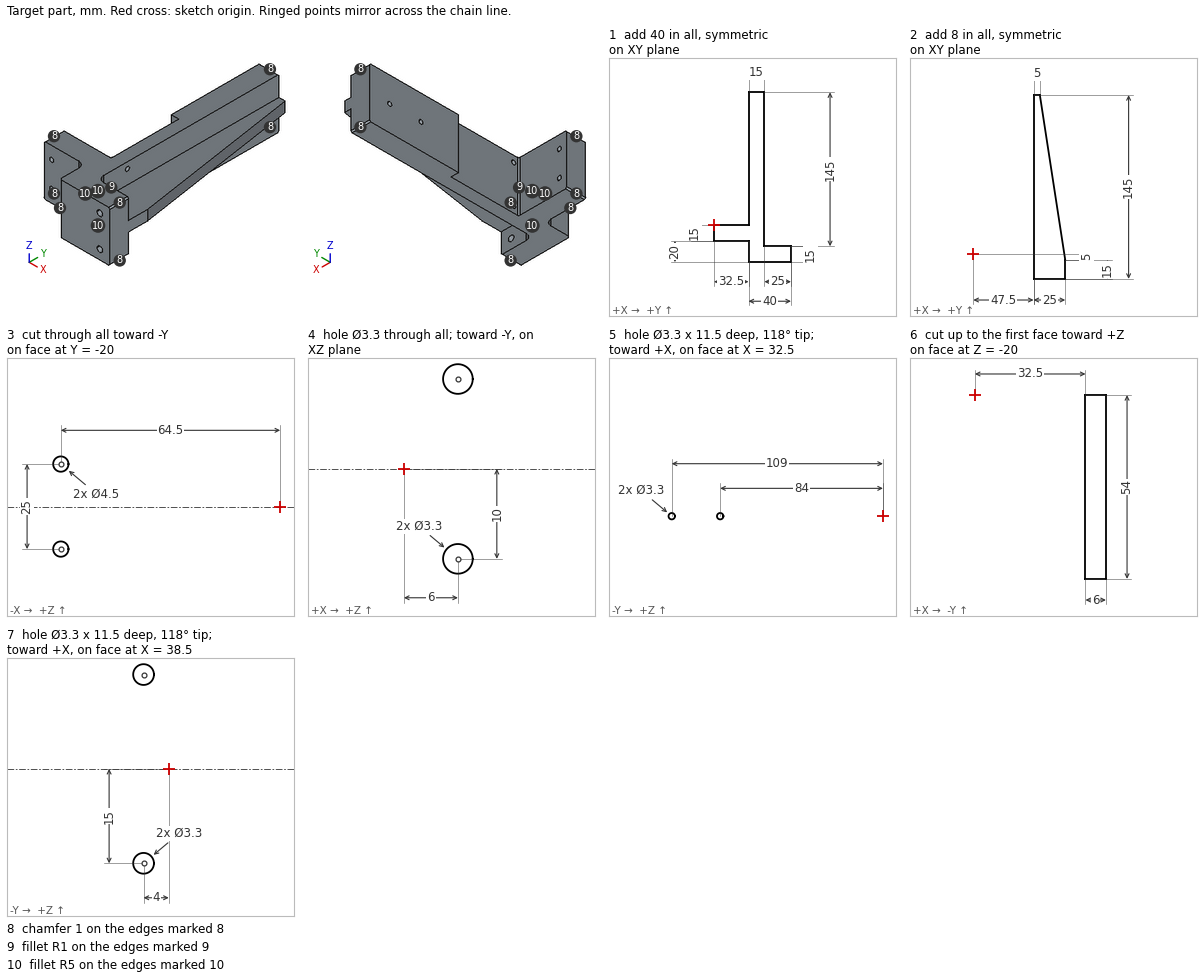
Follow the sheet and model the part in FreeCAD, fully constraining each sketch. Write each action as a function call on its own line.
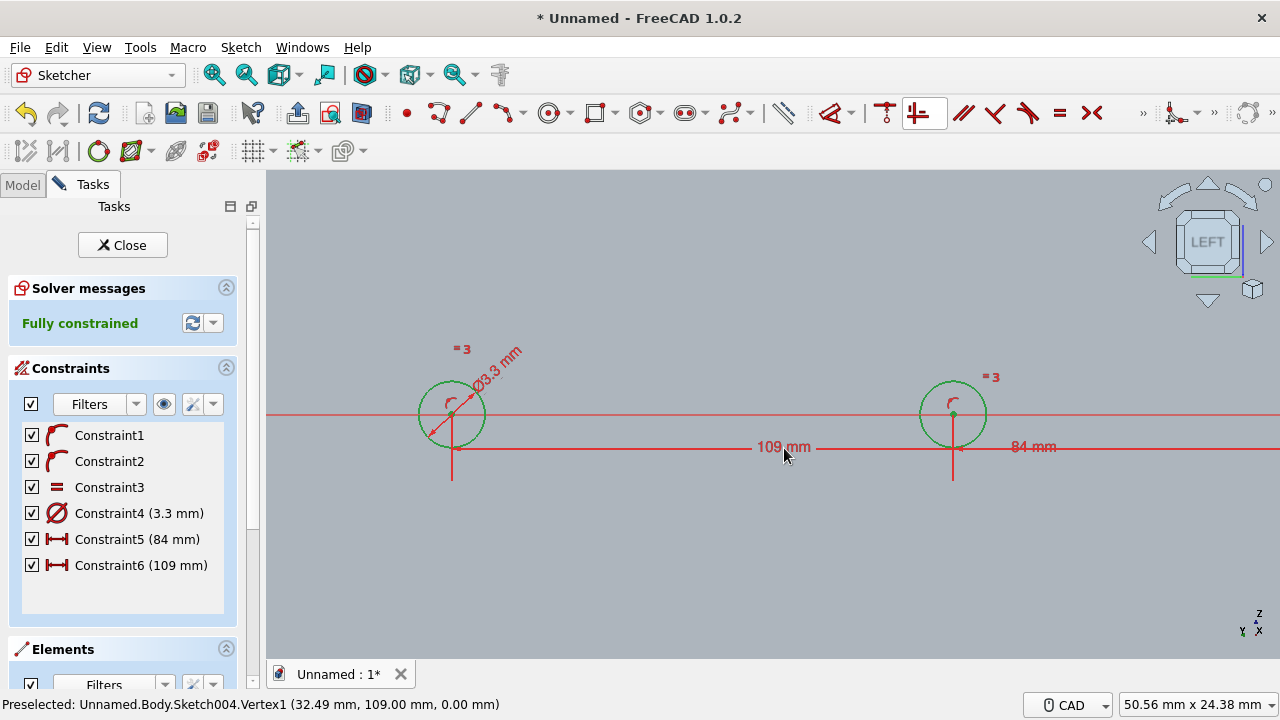
click(123, 245)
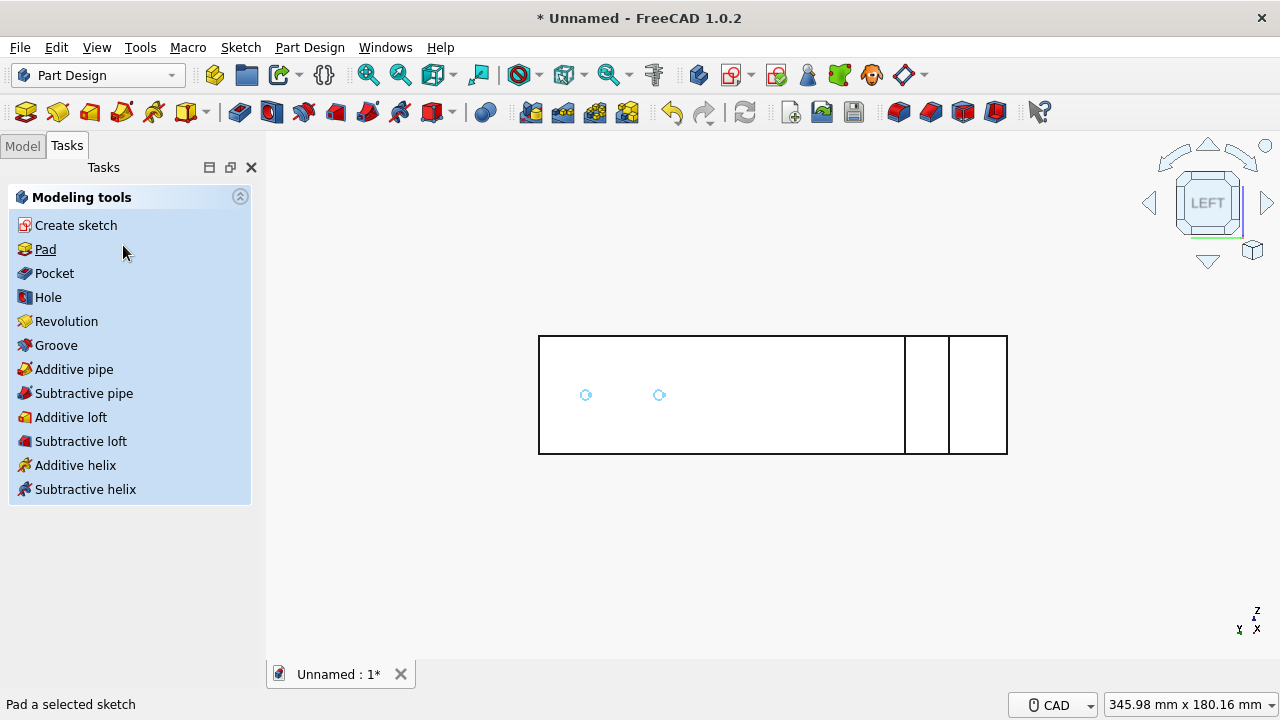
click(272, 112)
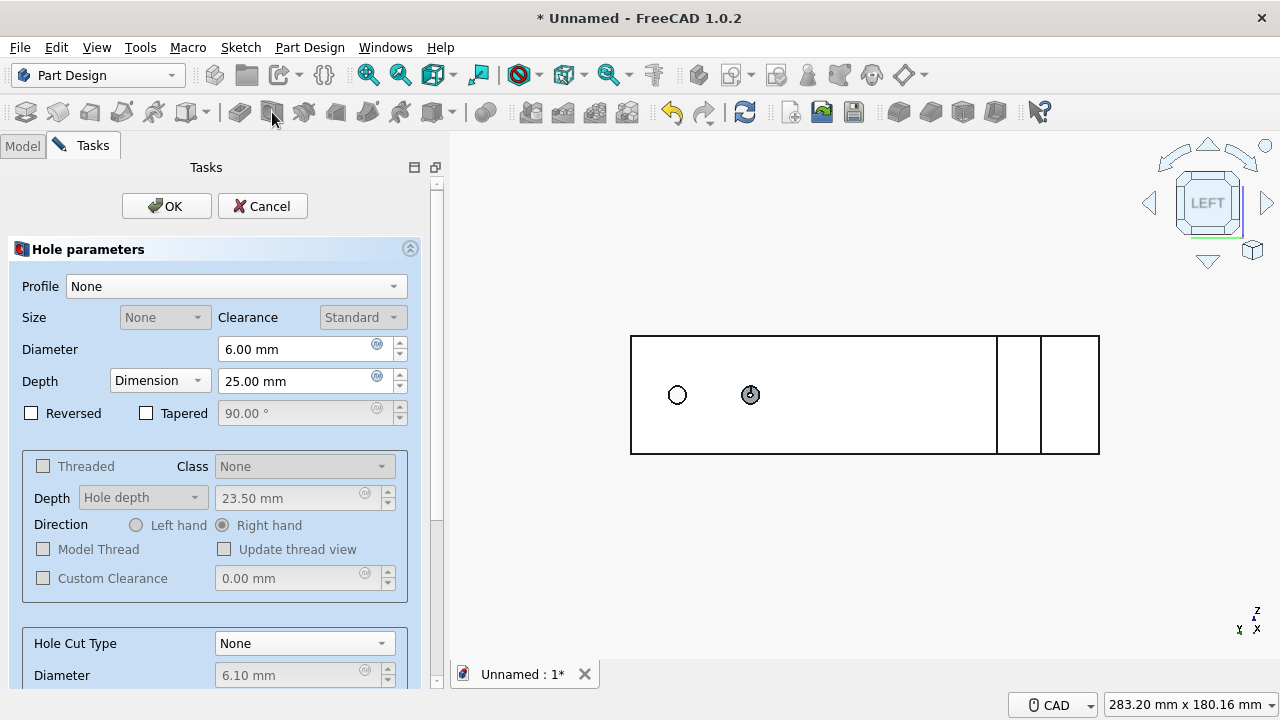
triple_click(305, 349)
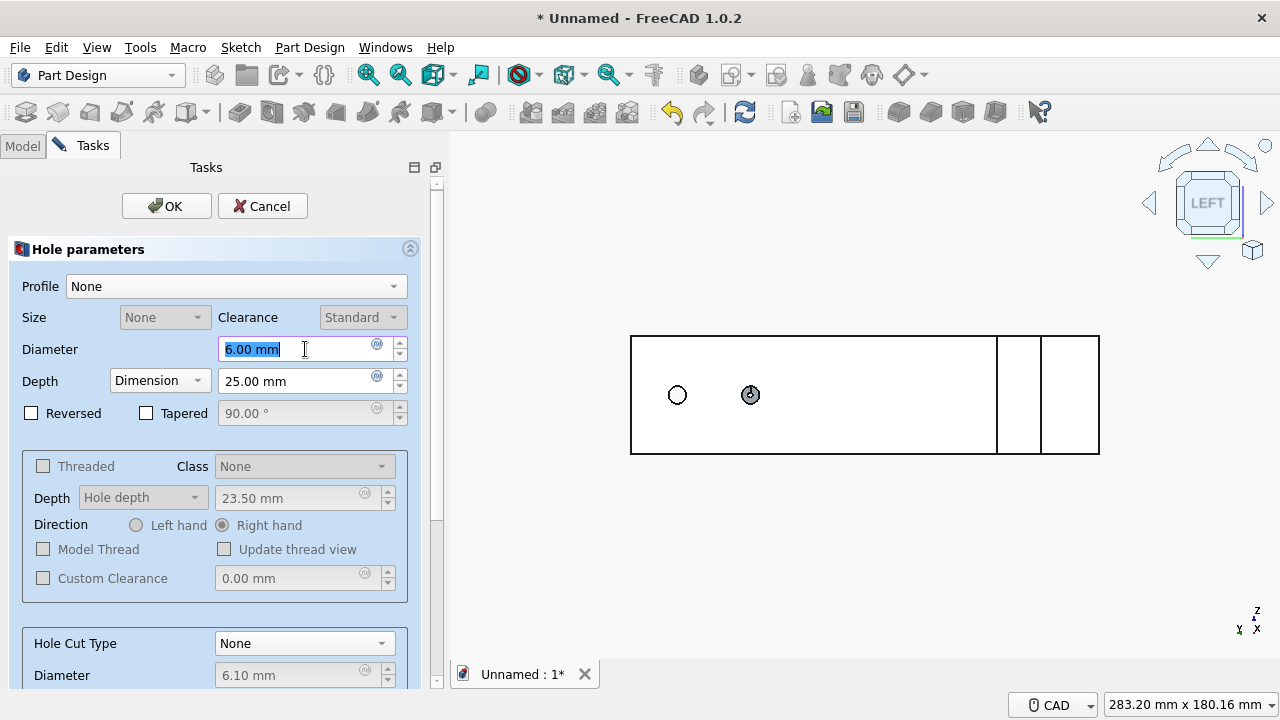
text(3.3)
key(Tab)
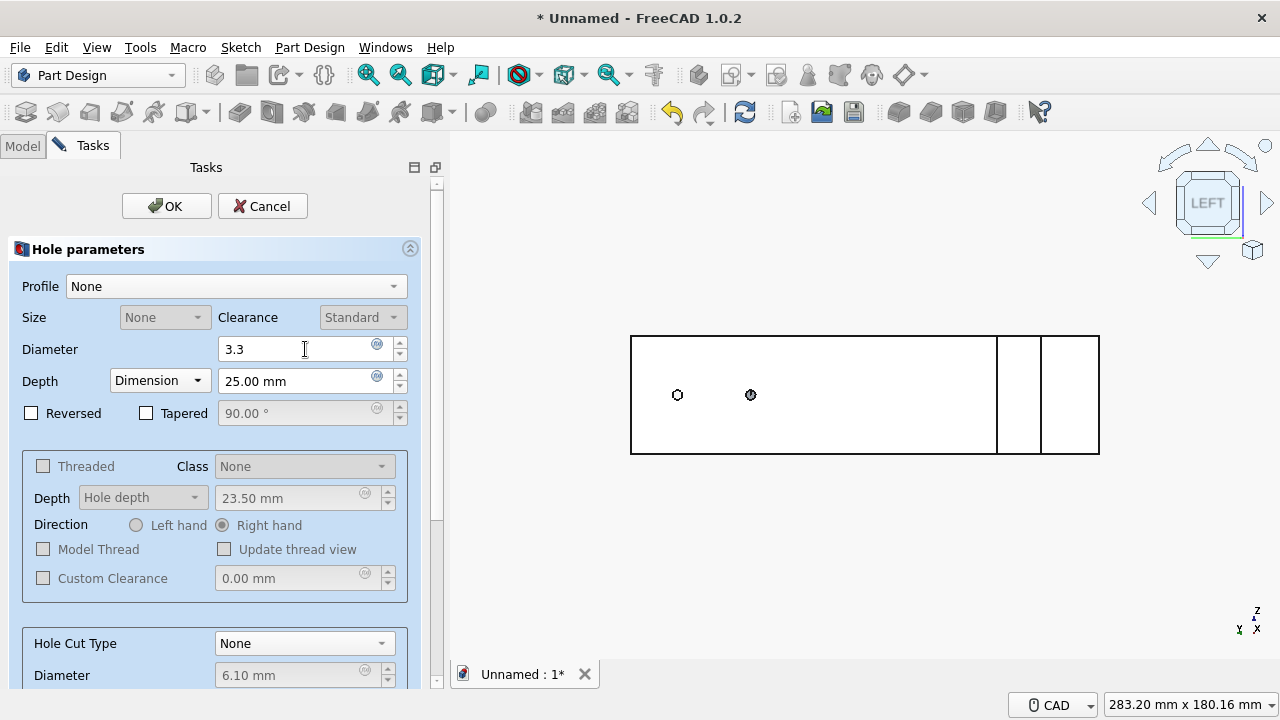
triple_click(305, 381)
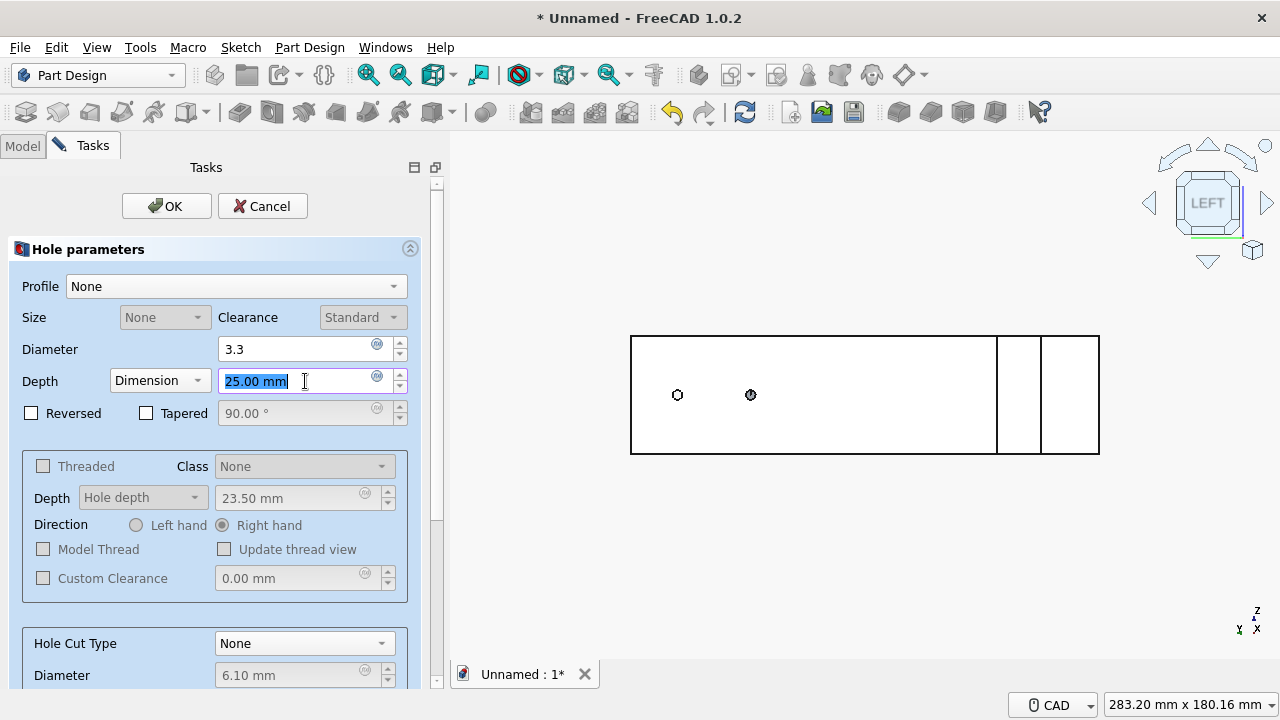
text(11.5)
key(Tab)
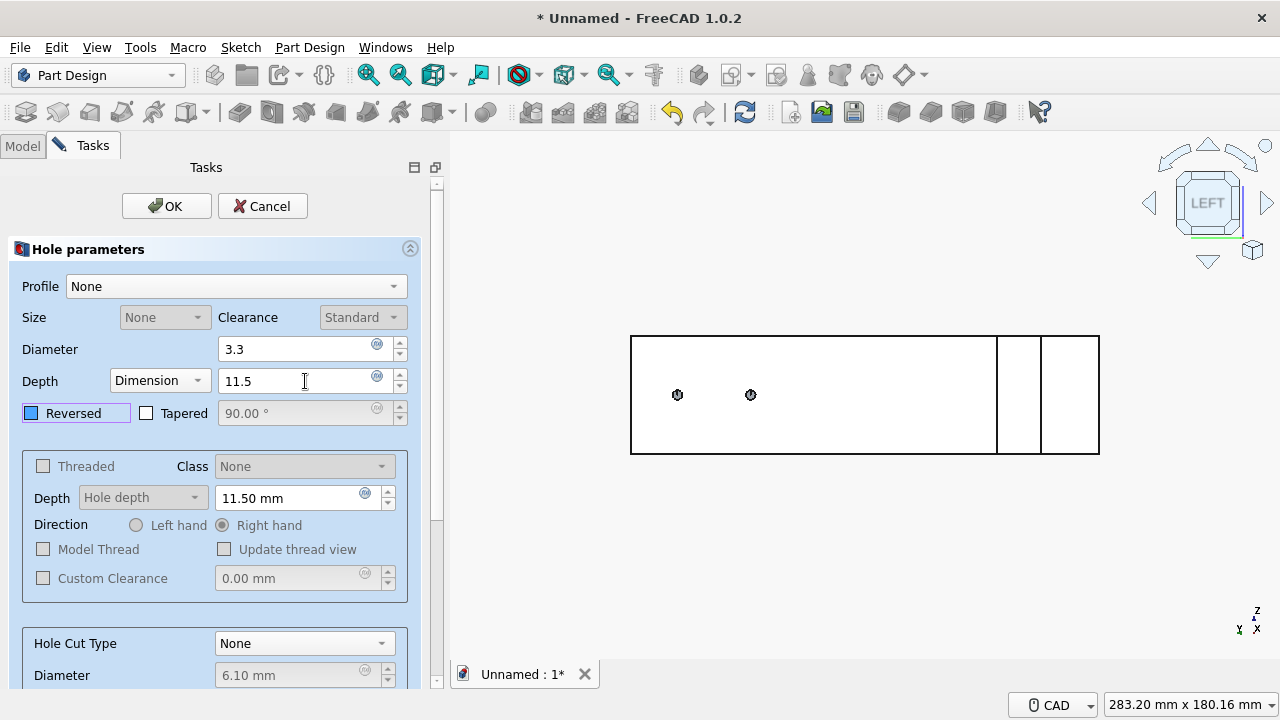
click(167, 206)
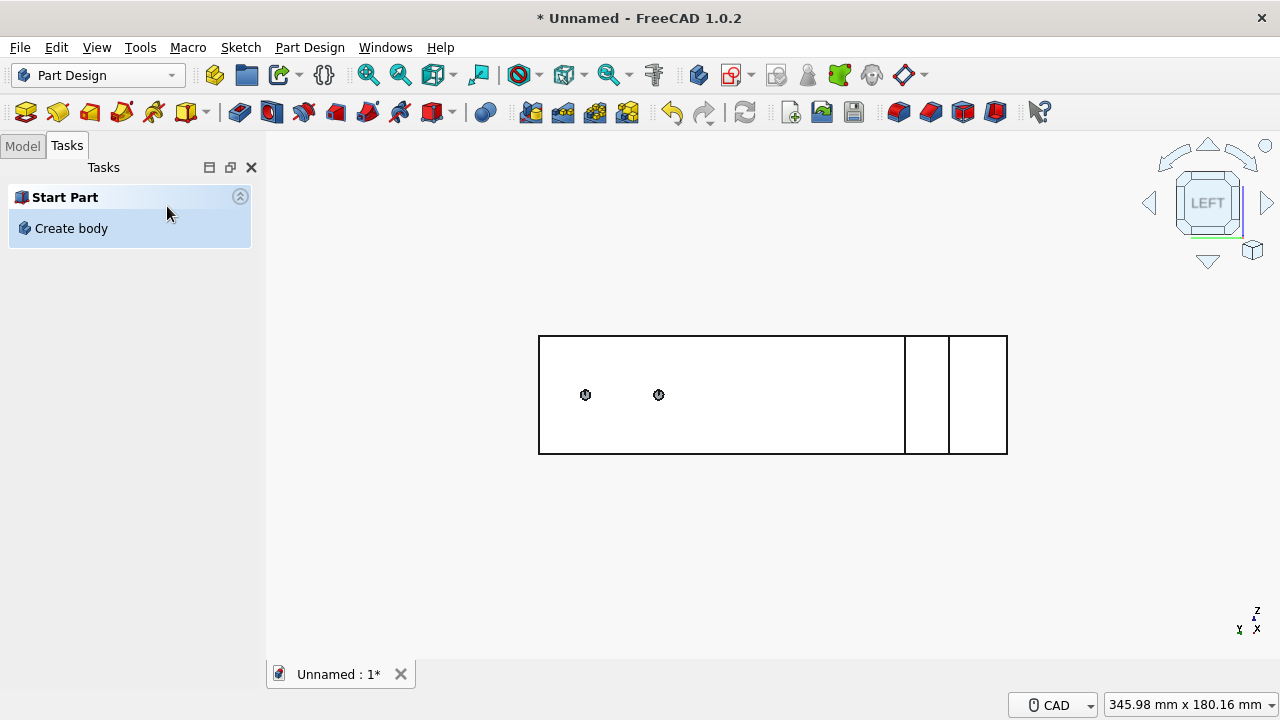
key(5)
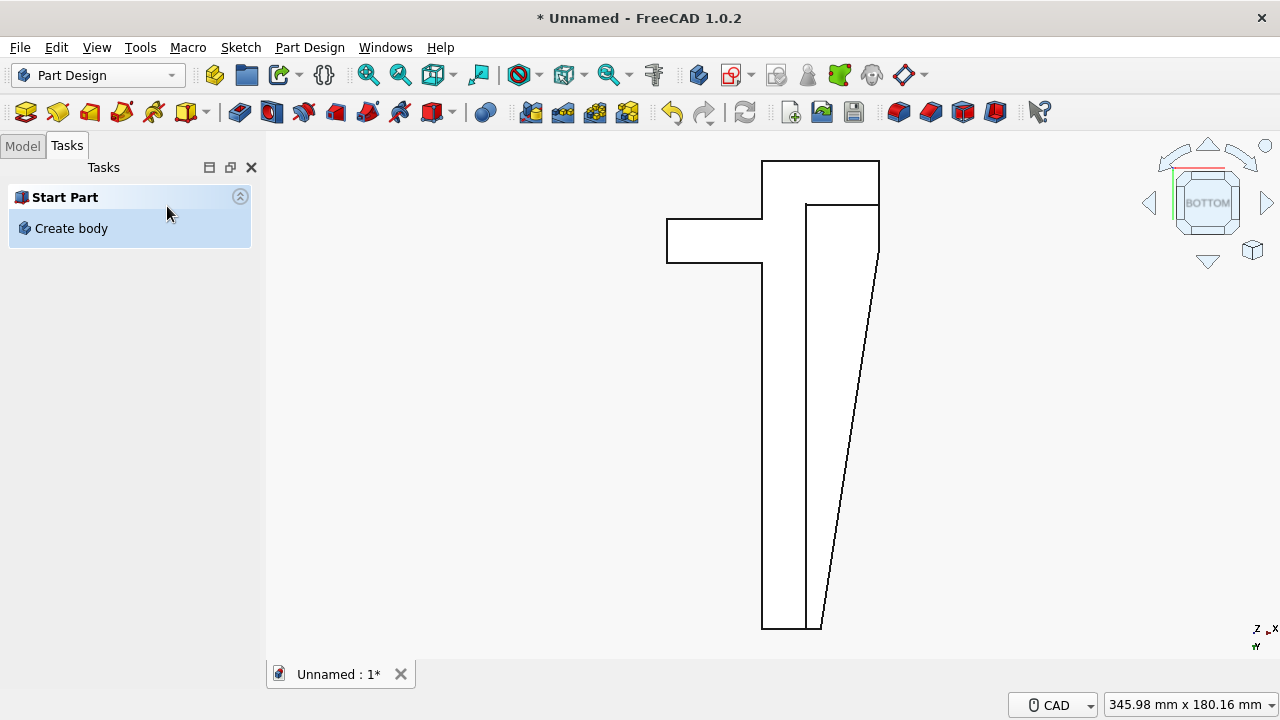
click(773, 260)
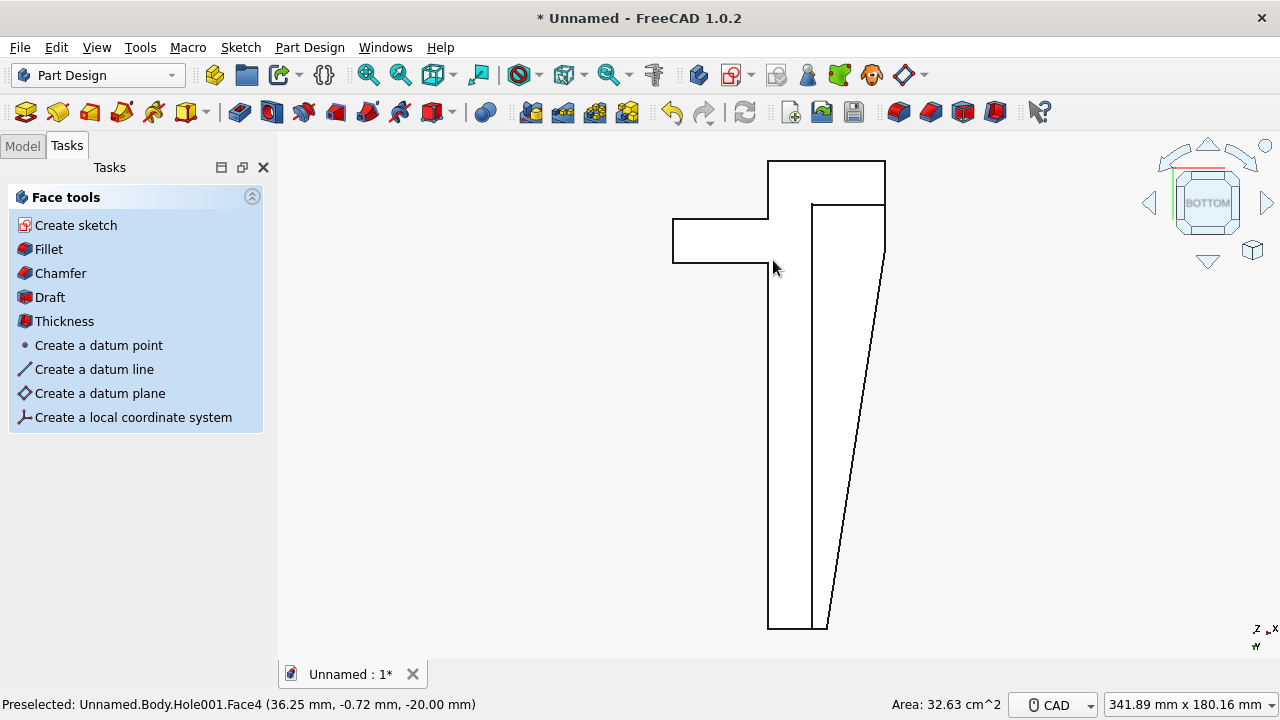
click(732, 76)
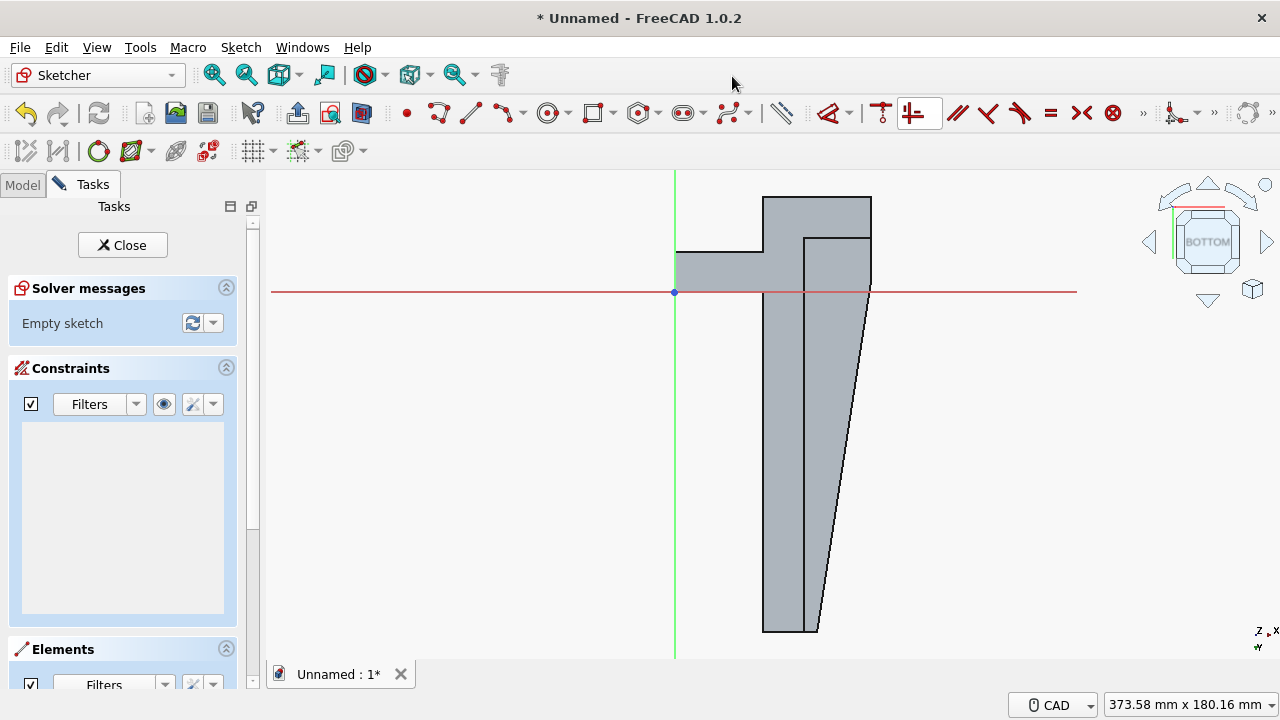
scroll(745, 326, up, 4)